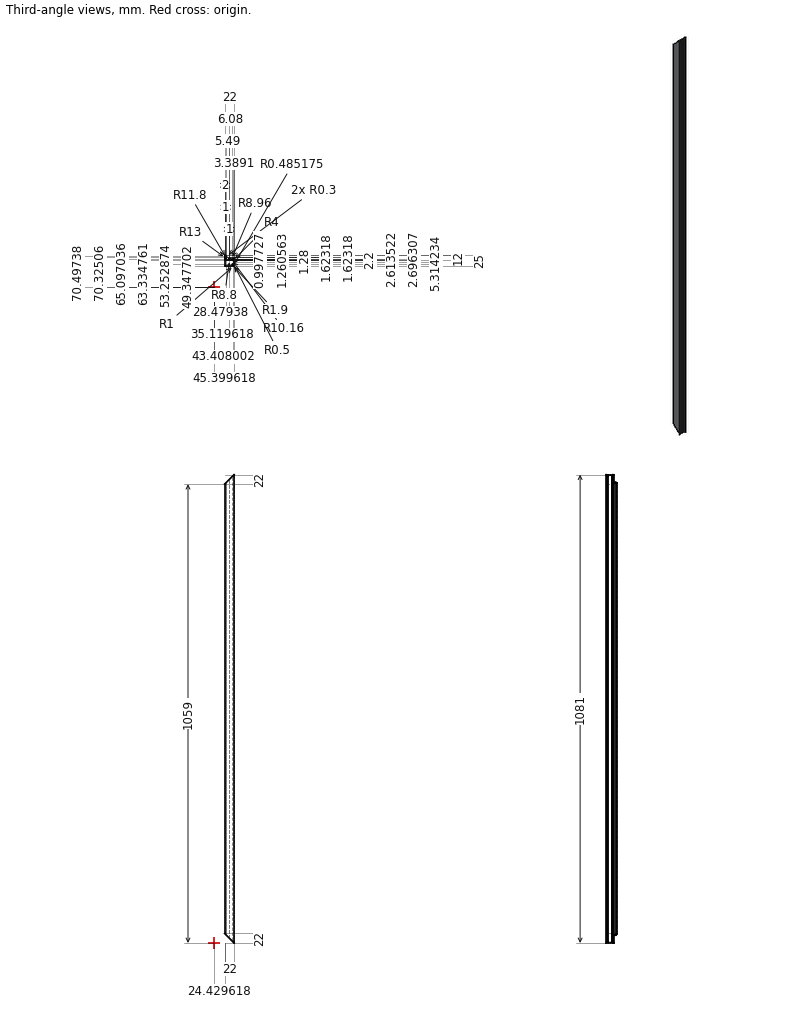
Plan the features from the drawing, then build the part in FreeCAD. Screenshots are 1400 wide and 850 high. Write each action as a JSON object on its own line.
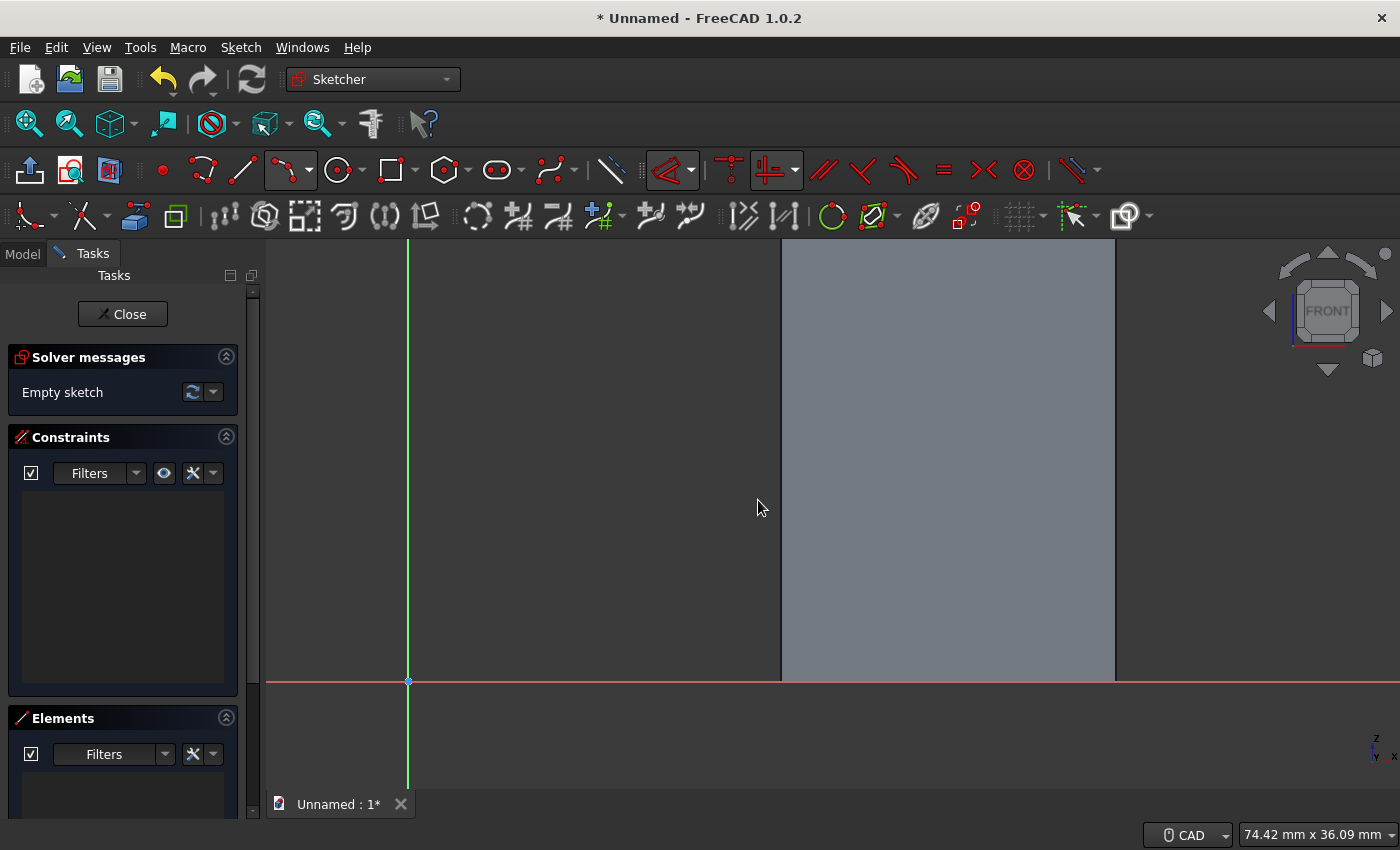
{"action": "left_click", "coordinate": [204, 170]}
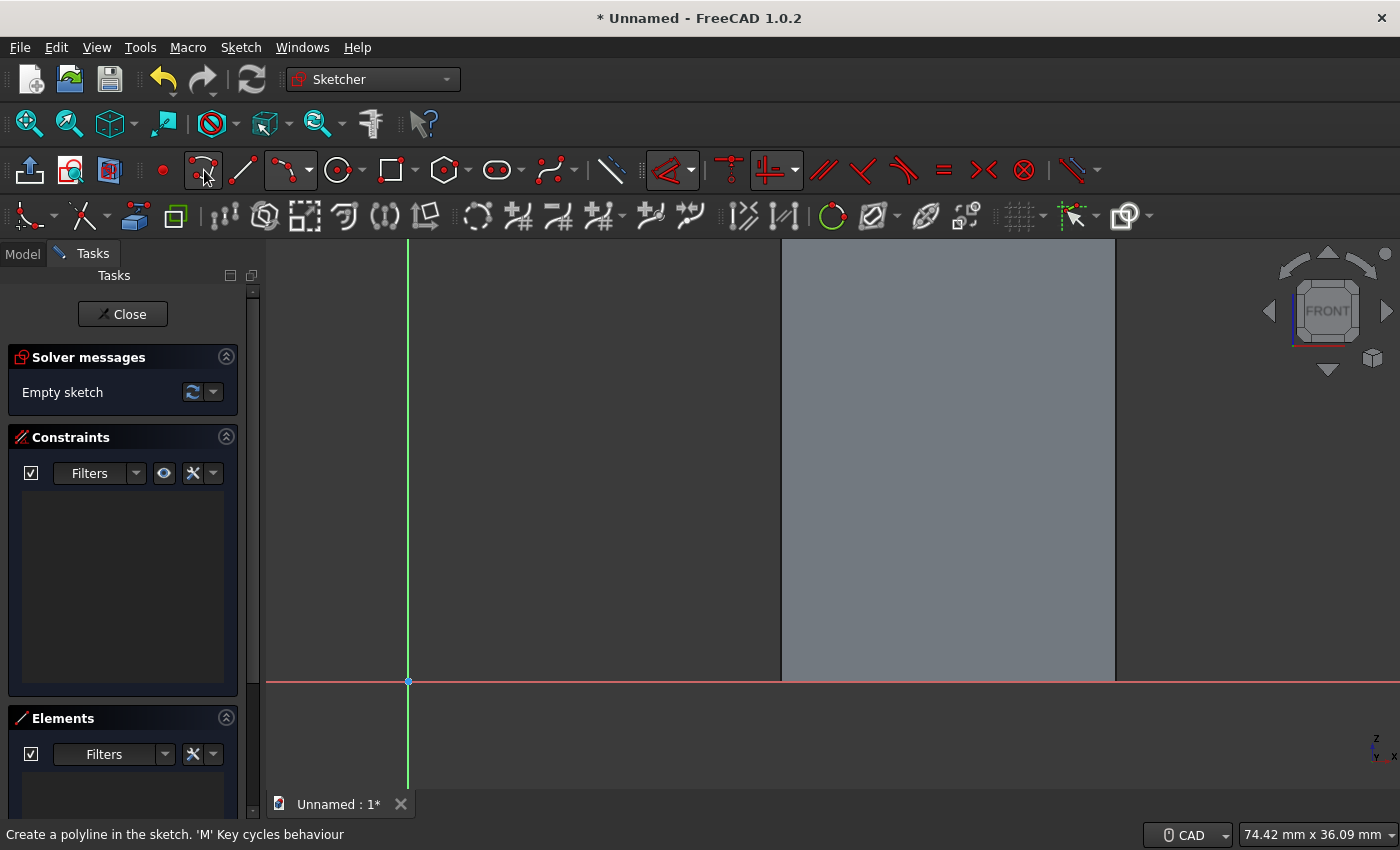
{"action": "left_click", "coordinate": [781, 682]}
{"action": "left_click", "coordinate": [1116, 673]}
{"action": "left_click", "coordinate": [781, 346]}
{"action": "left_click", "coordinate": [781, 682]}
{"action": "key", "text": "Escape"}
{"action": "key", "text": "Escape"}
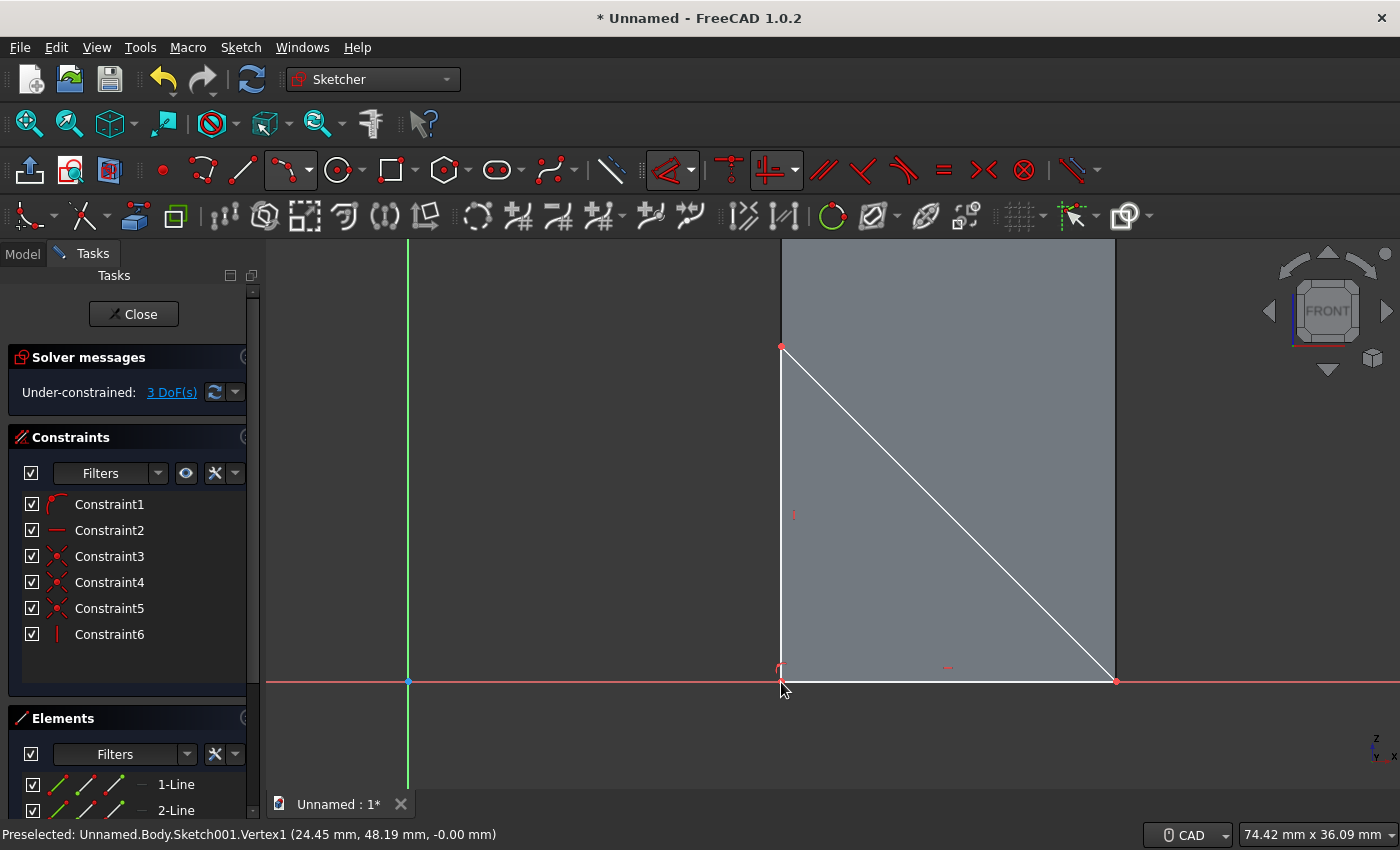
{"action": "left_click", "coordinate": [882, 682]}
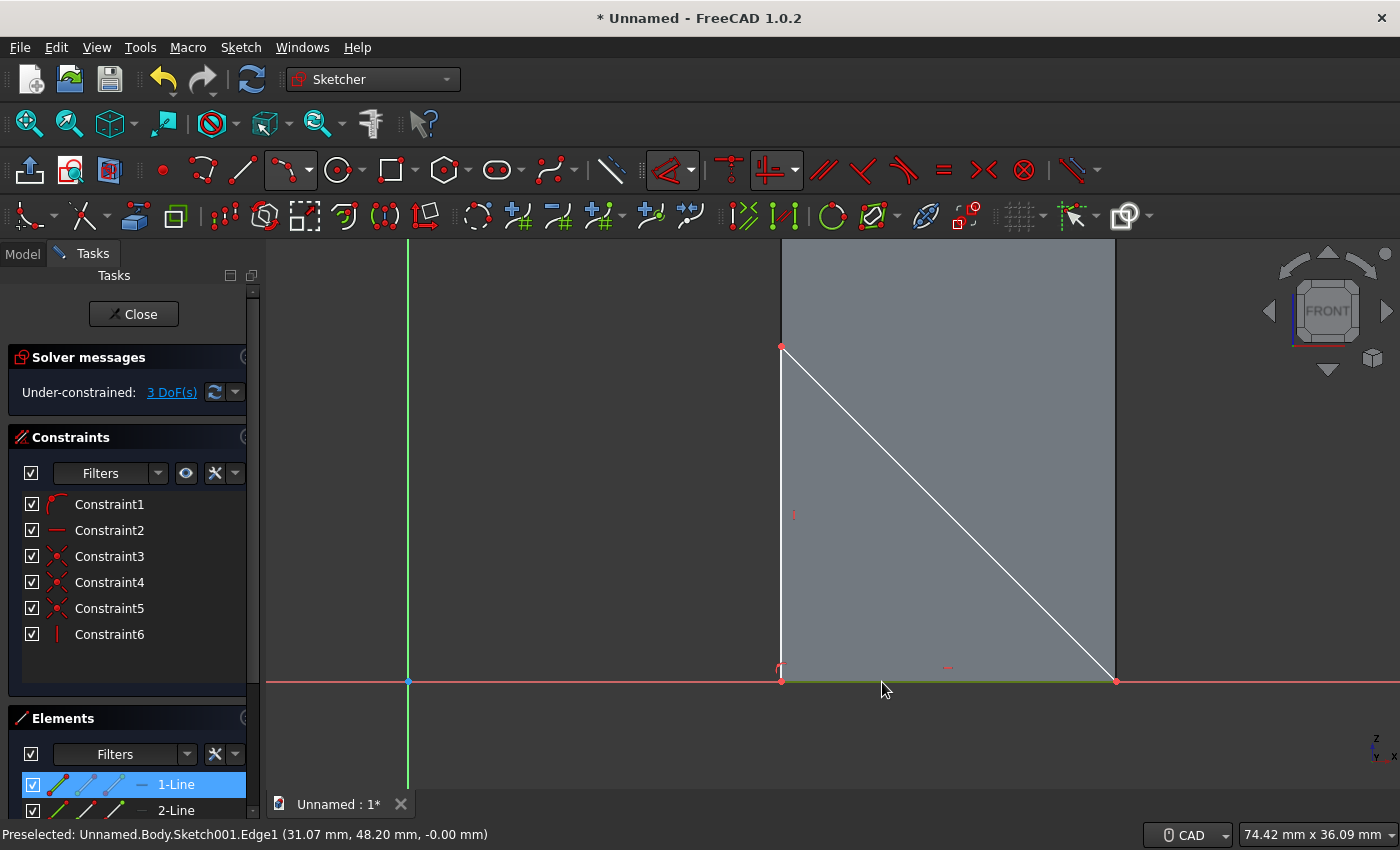
{"action": "left_click", "coordinate": [694, 170]}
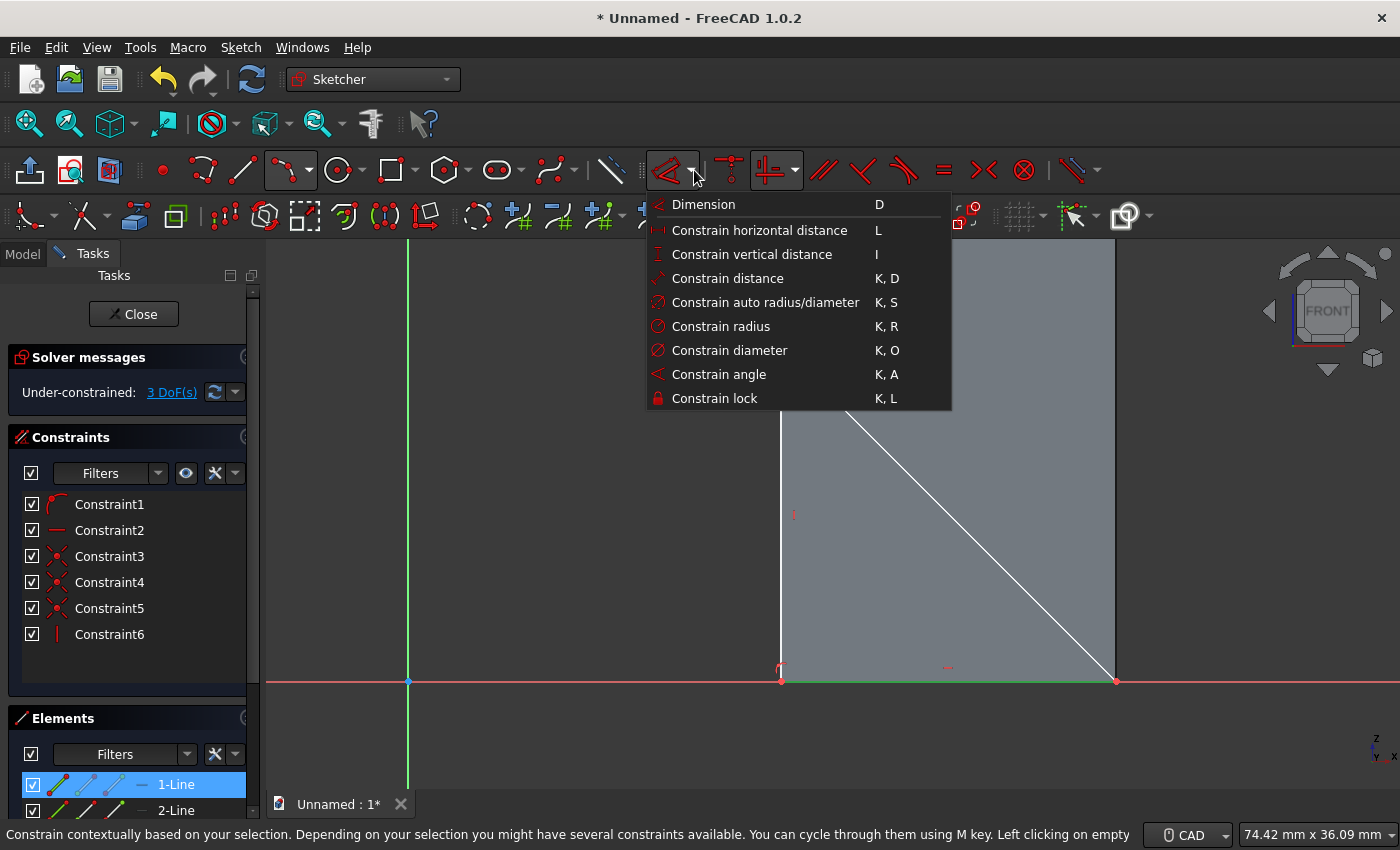
{"action": "left_click", "coordinate": [799, 230]}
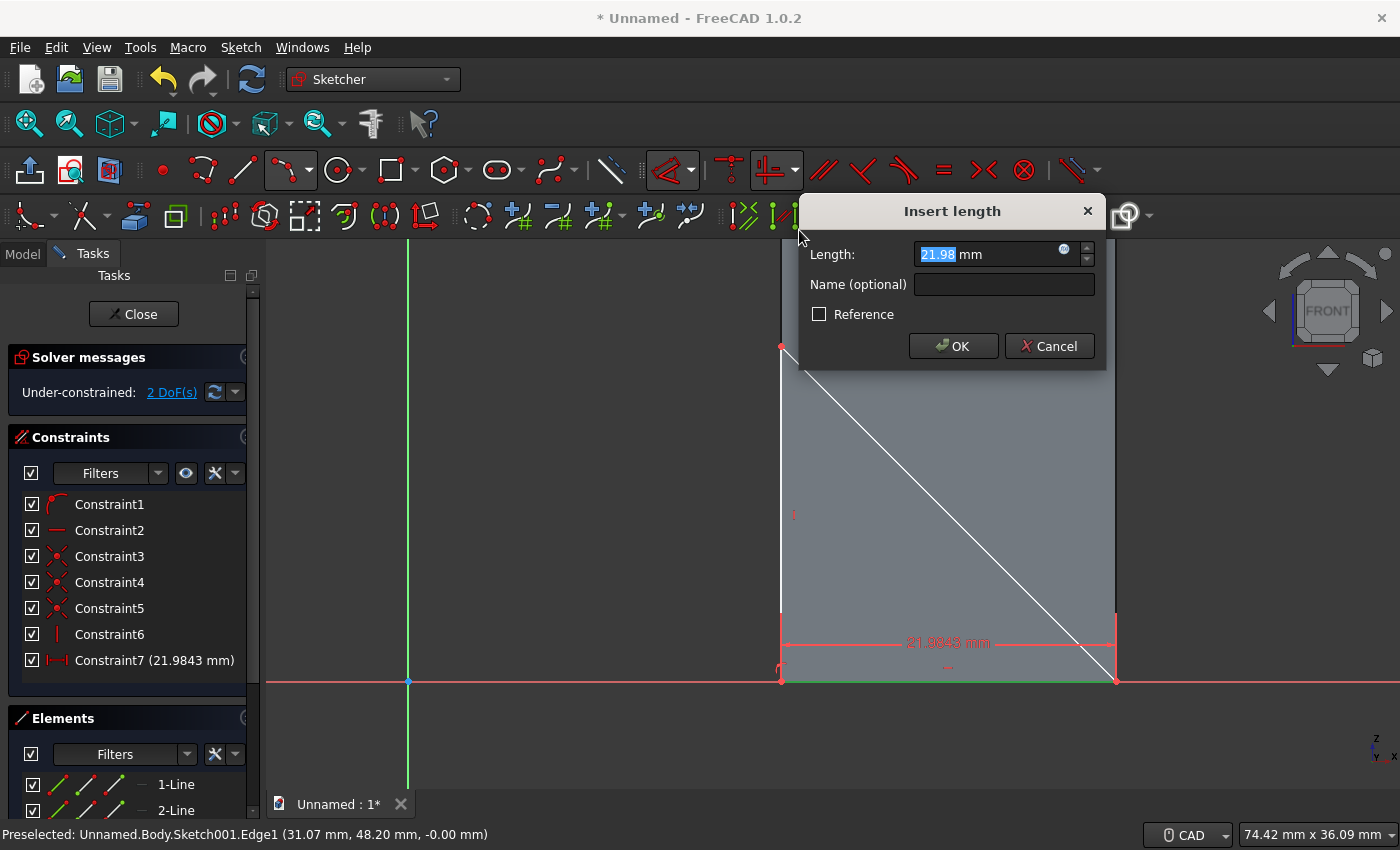
{"action": "type", "text": "22"}
{"action": "key", "text": "Return"}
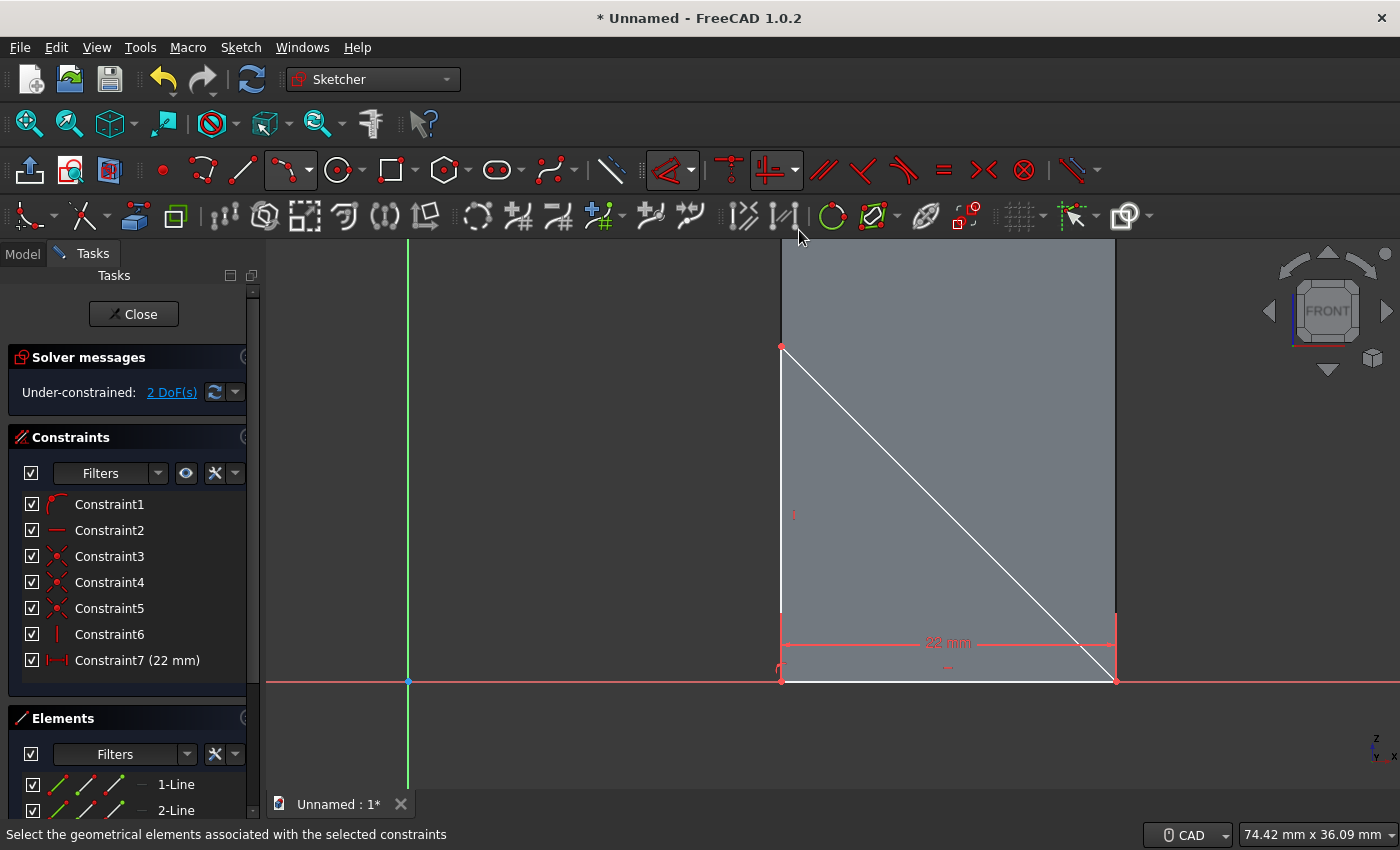
{"action": "left_click", "coordinate": [781, 447]}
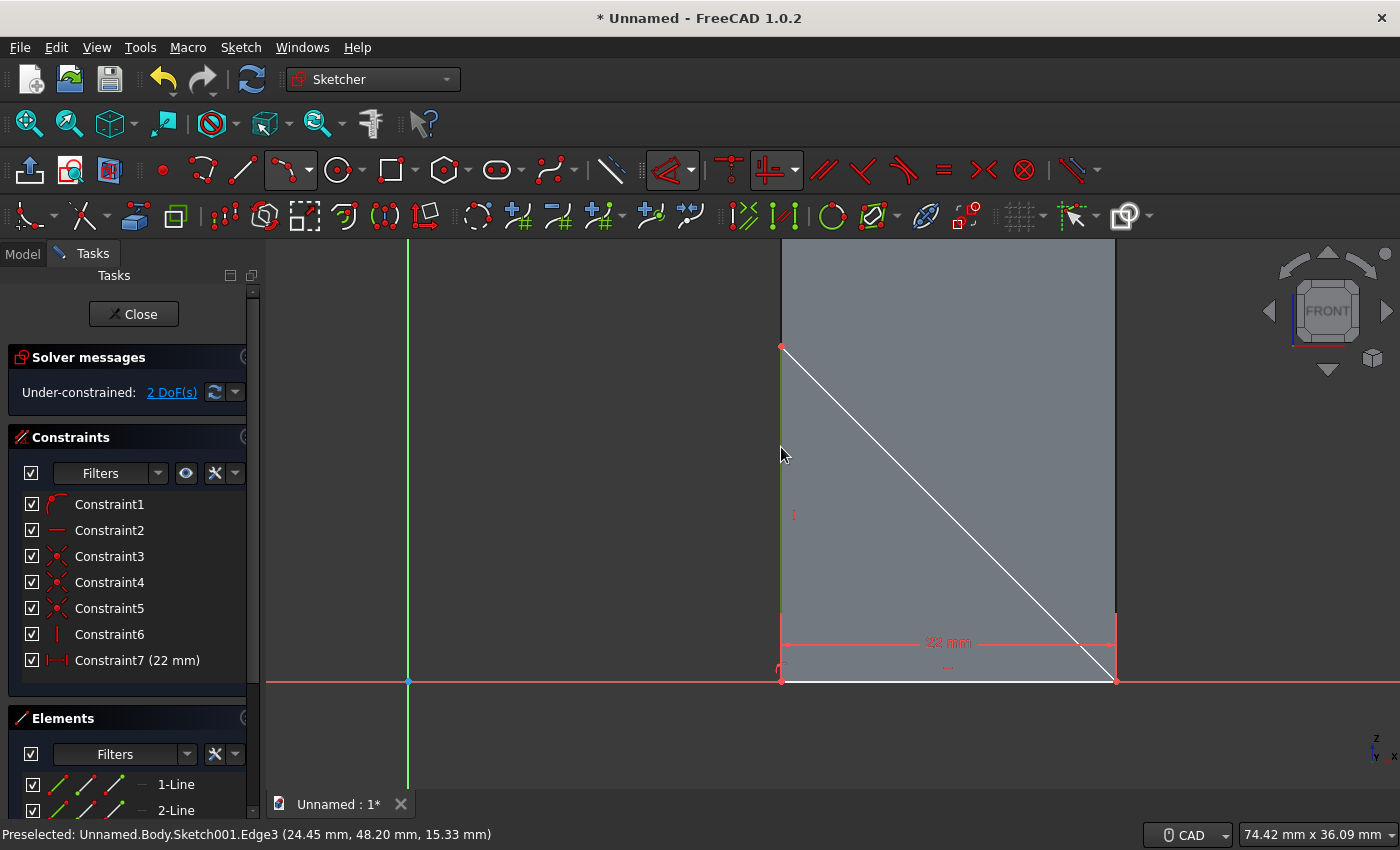
{"action": "key", "text": "i"}